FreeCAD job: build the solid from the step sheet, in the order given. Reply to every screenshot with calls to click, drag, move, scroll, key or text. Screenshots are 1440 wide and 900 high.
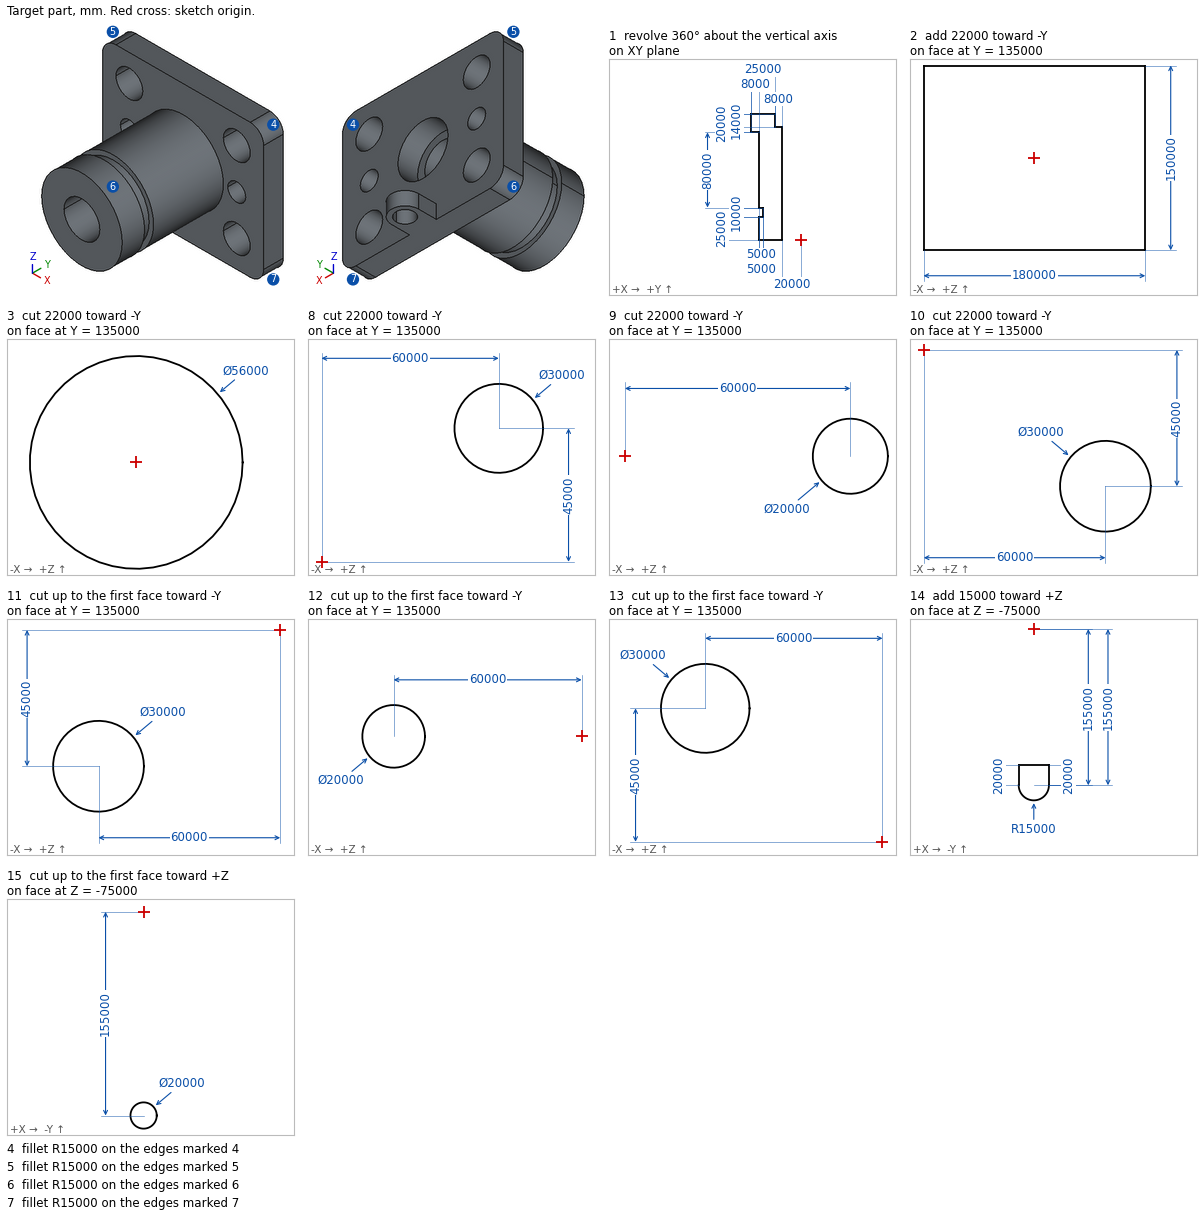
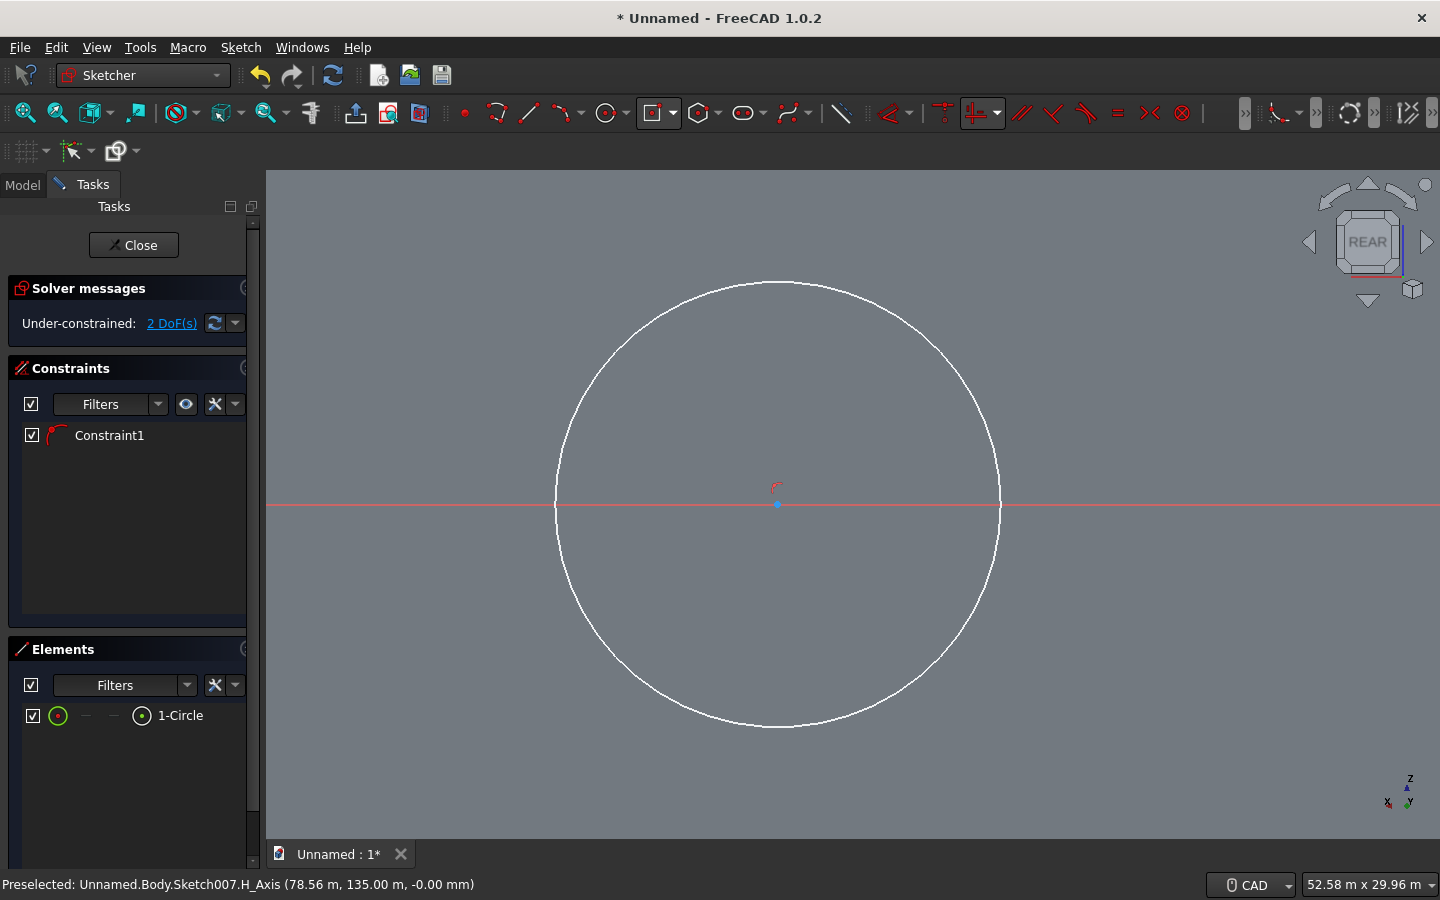
key(d)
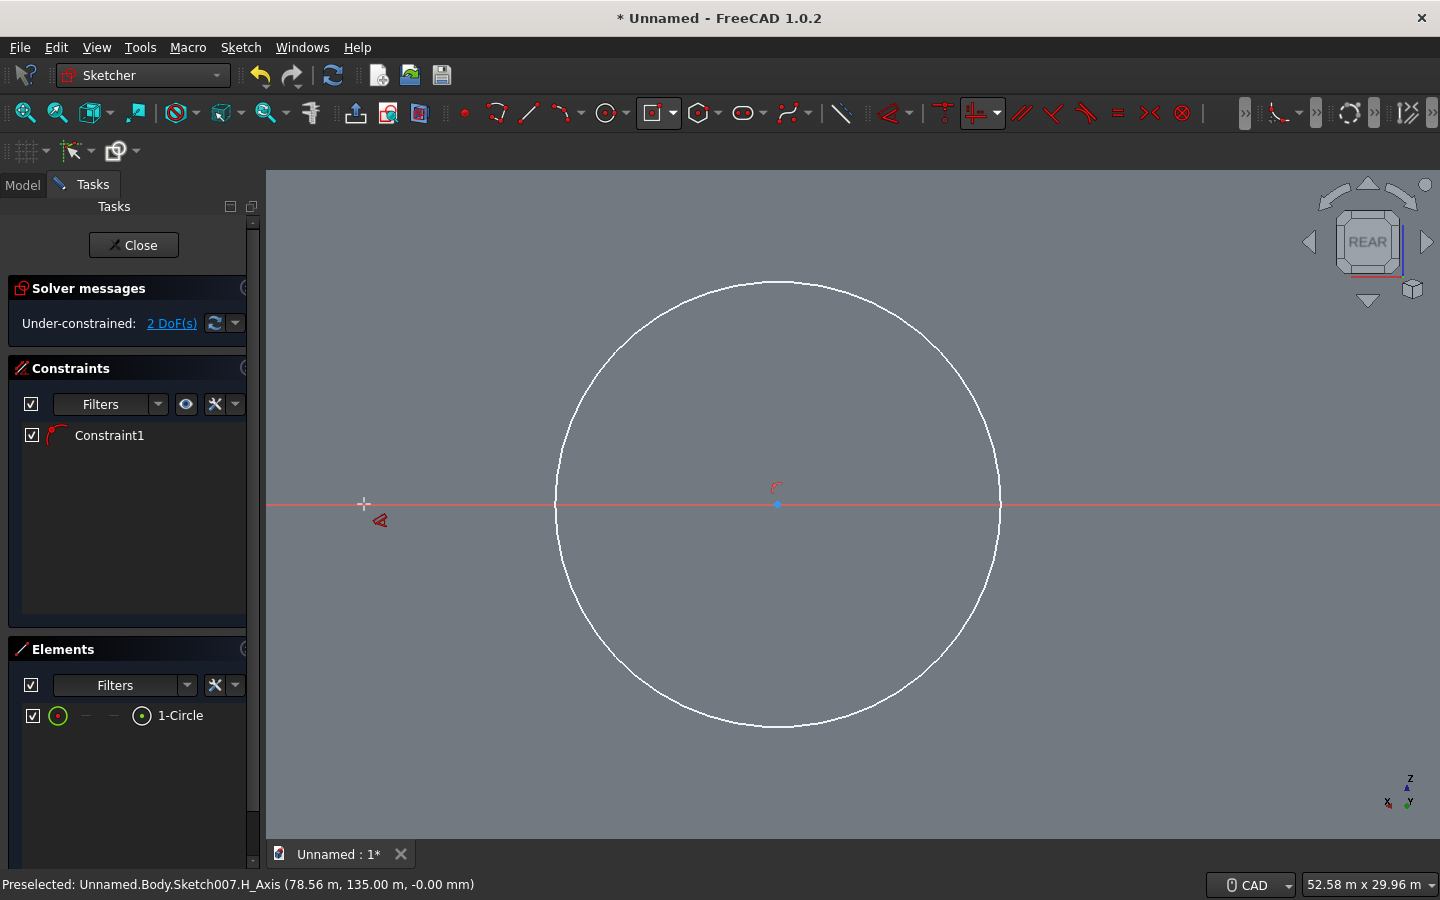
click(935, 347)
click(958, 324)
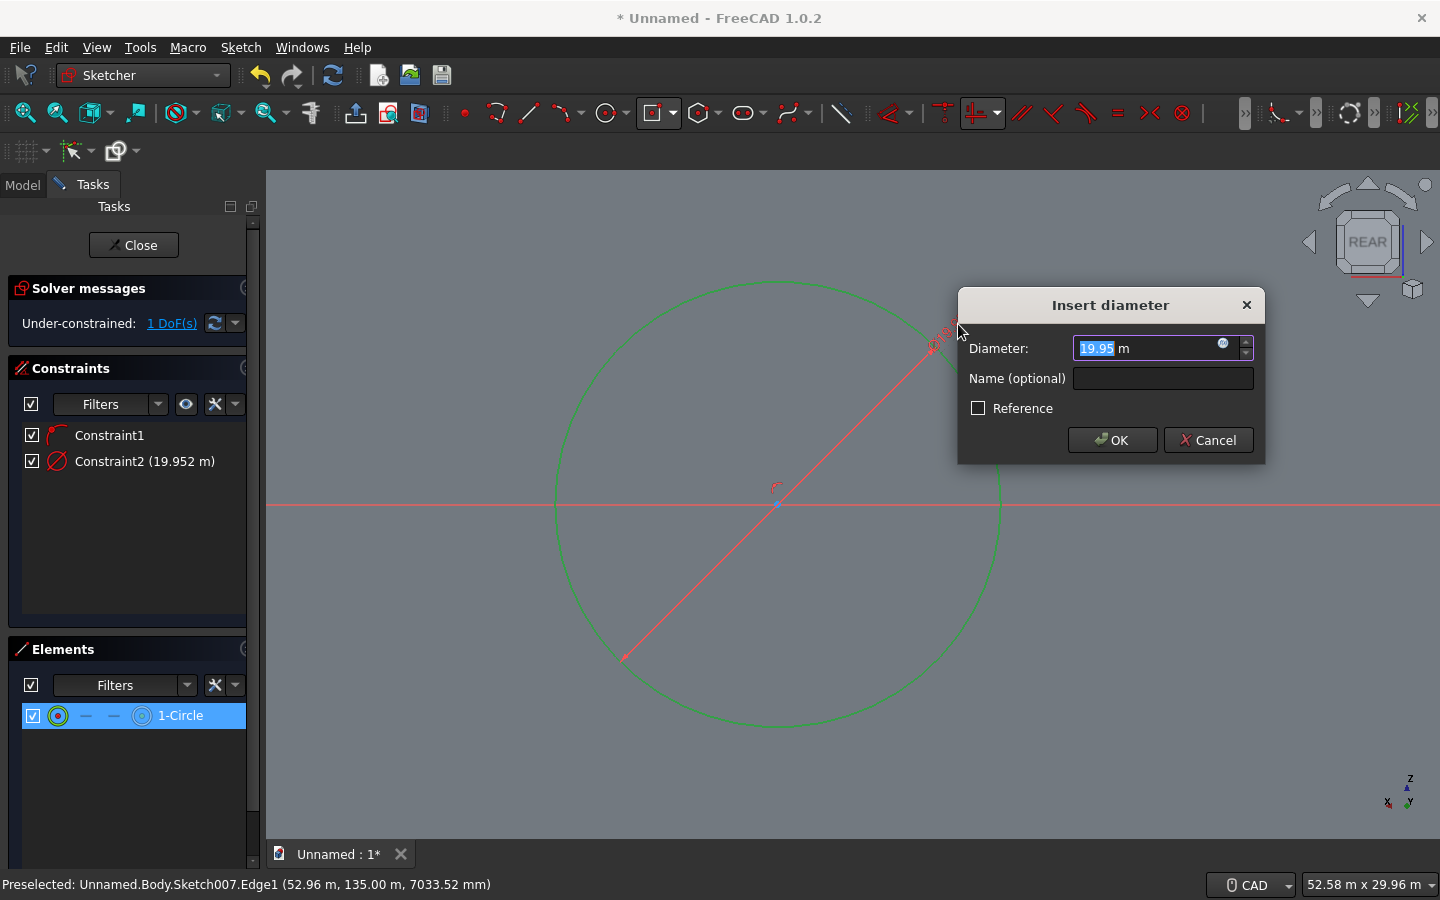
key(ctrl+a)
text(20000 mm)
key(Return)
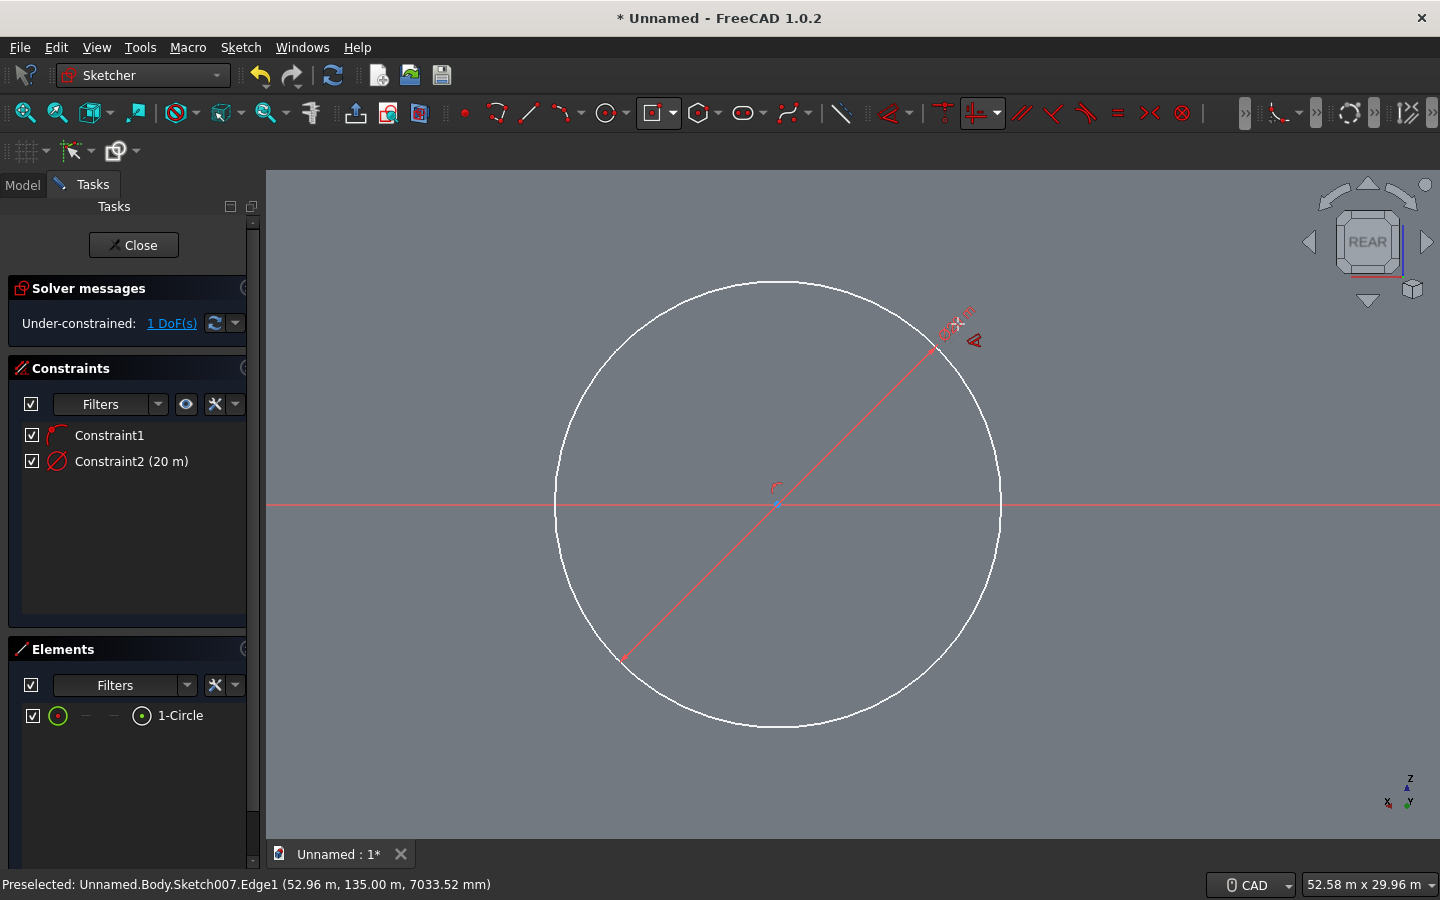
click(778, 504)
click(1026, 538)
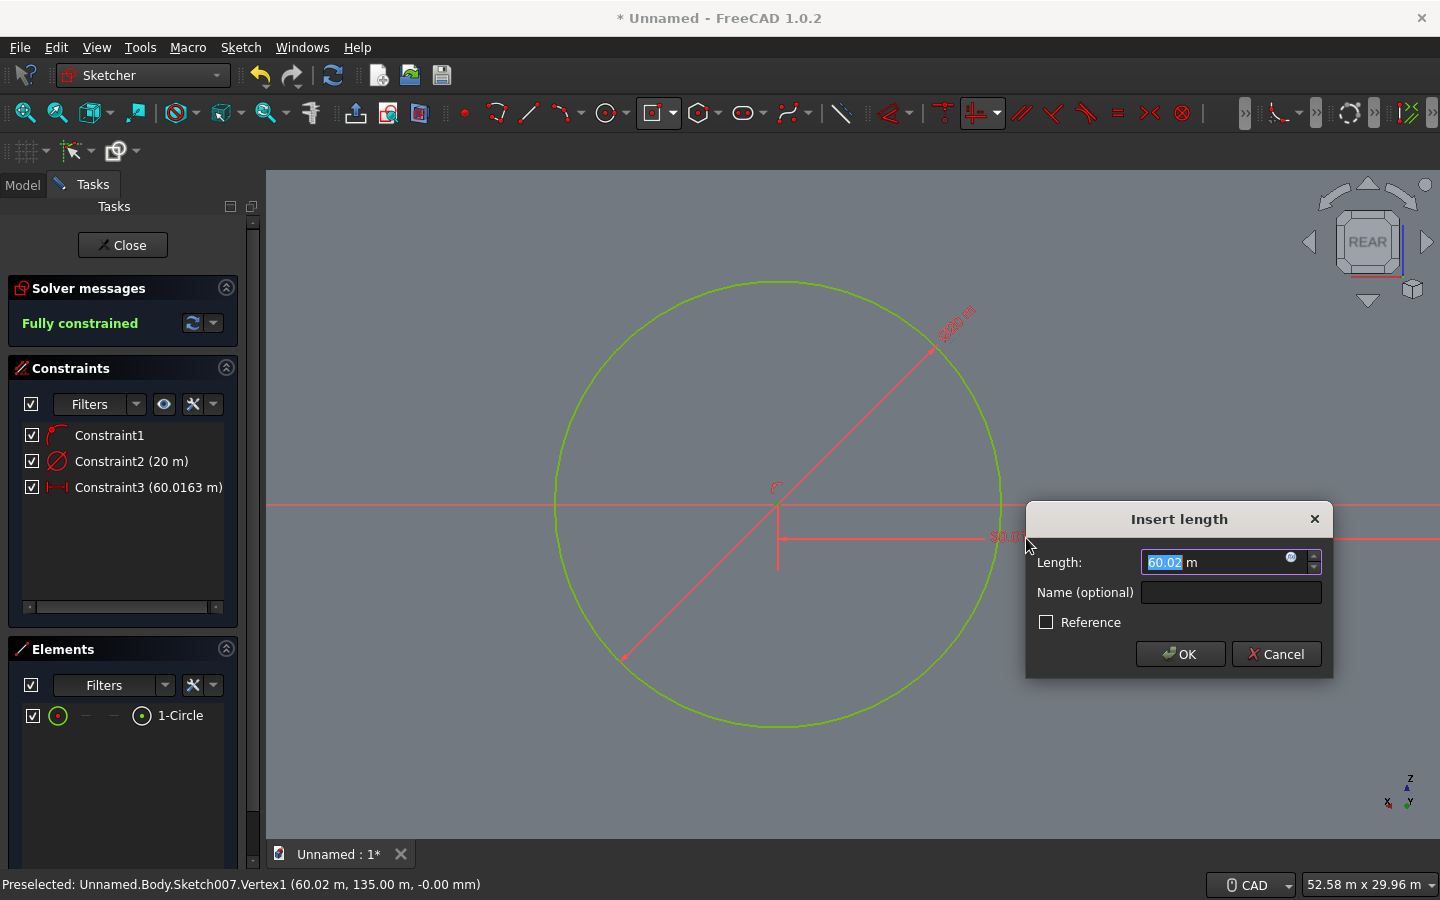
key(ctrl+a)
text(60000 mm)
key(Return)
key(Escape)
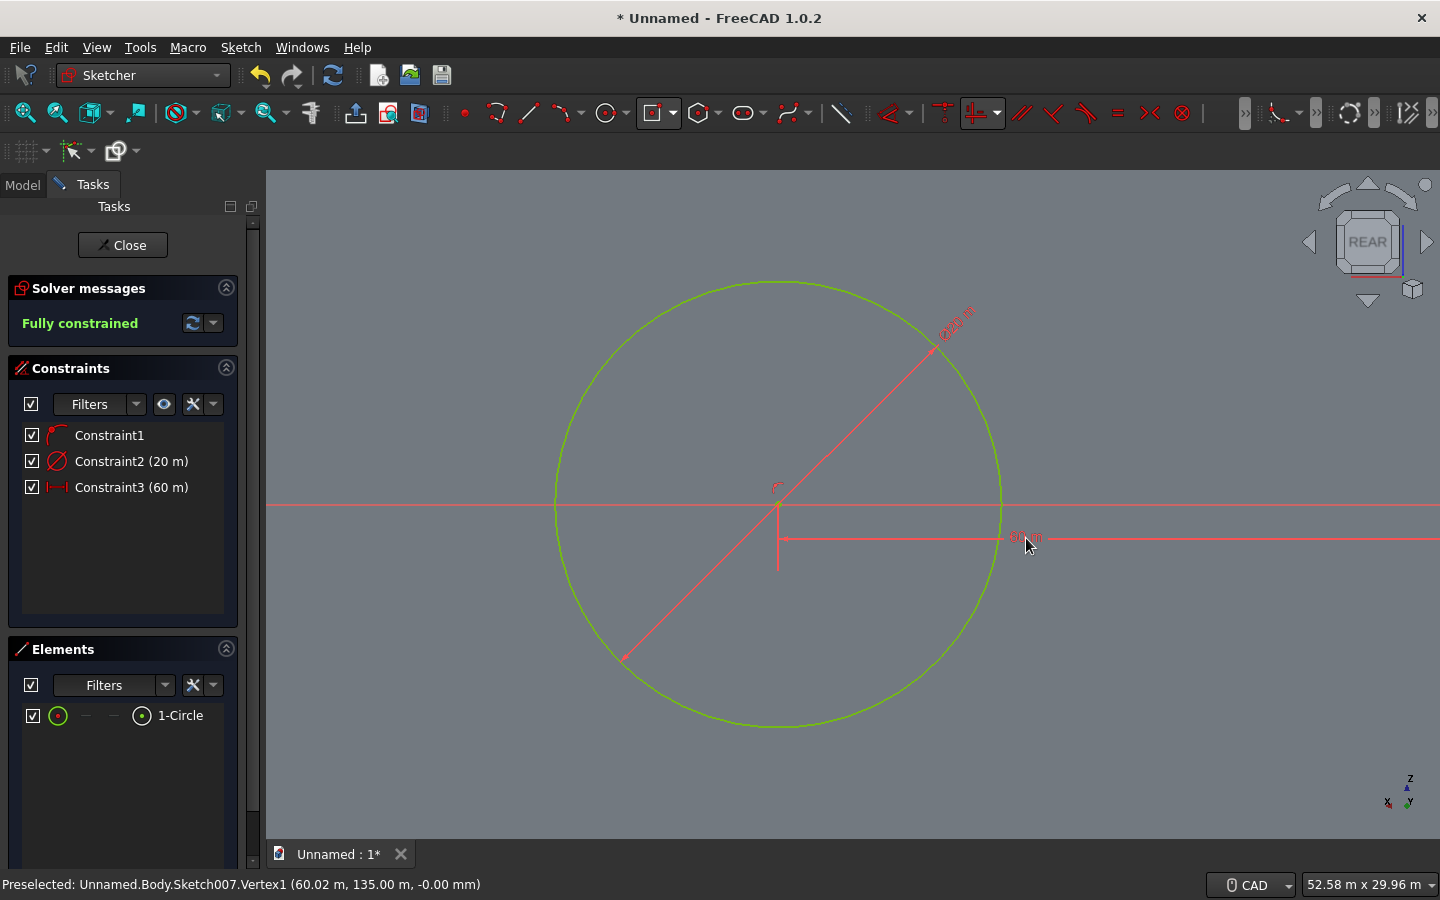
click(123, 245)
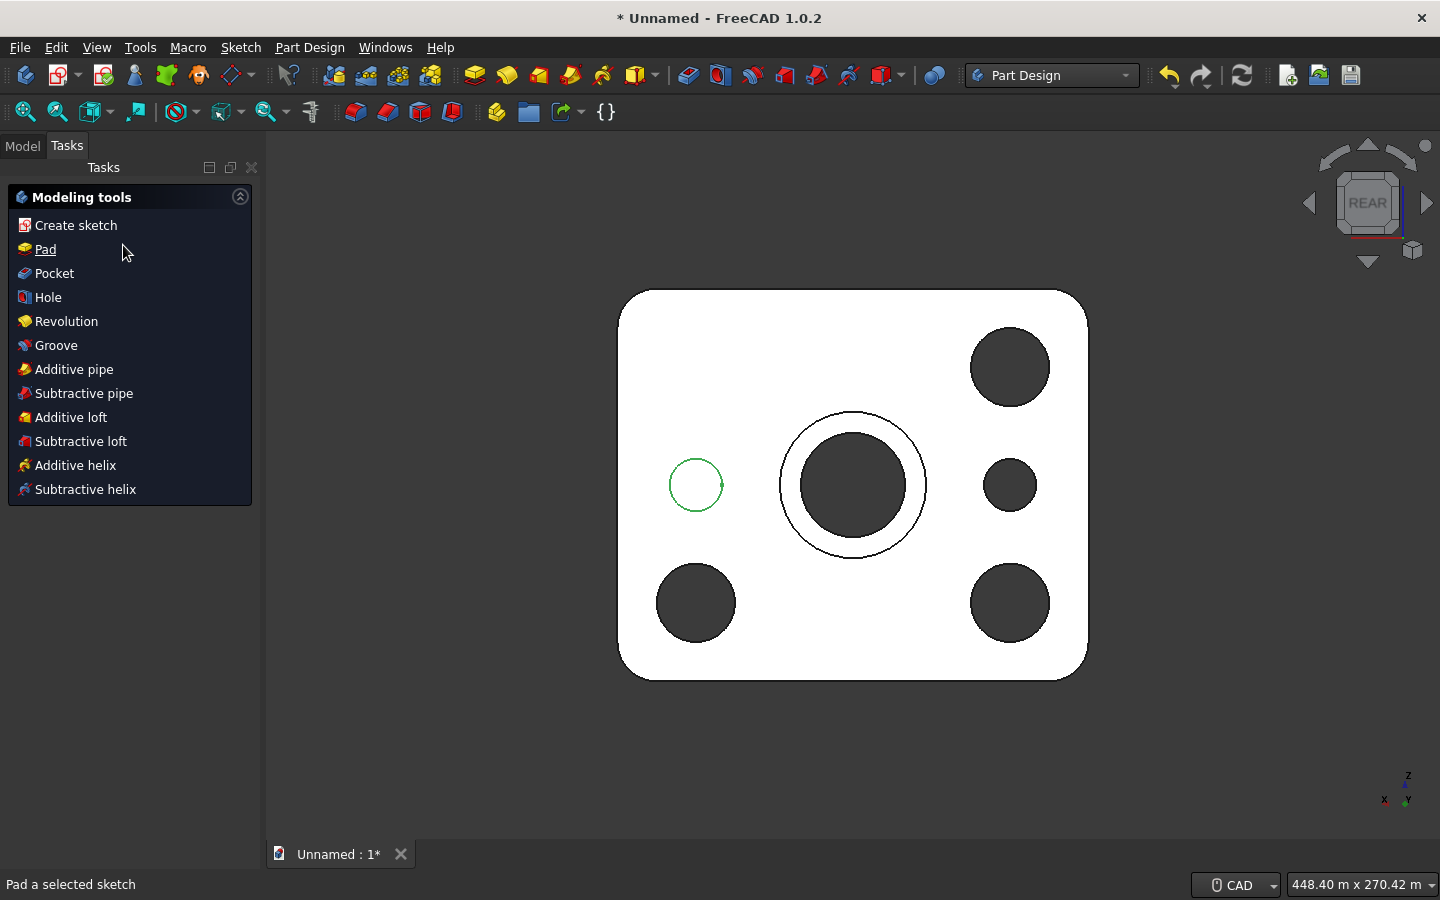
click(690, 76)